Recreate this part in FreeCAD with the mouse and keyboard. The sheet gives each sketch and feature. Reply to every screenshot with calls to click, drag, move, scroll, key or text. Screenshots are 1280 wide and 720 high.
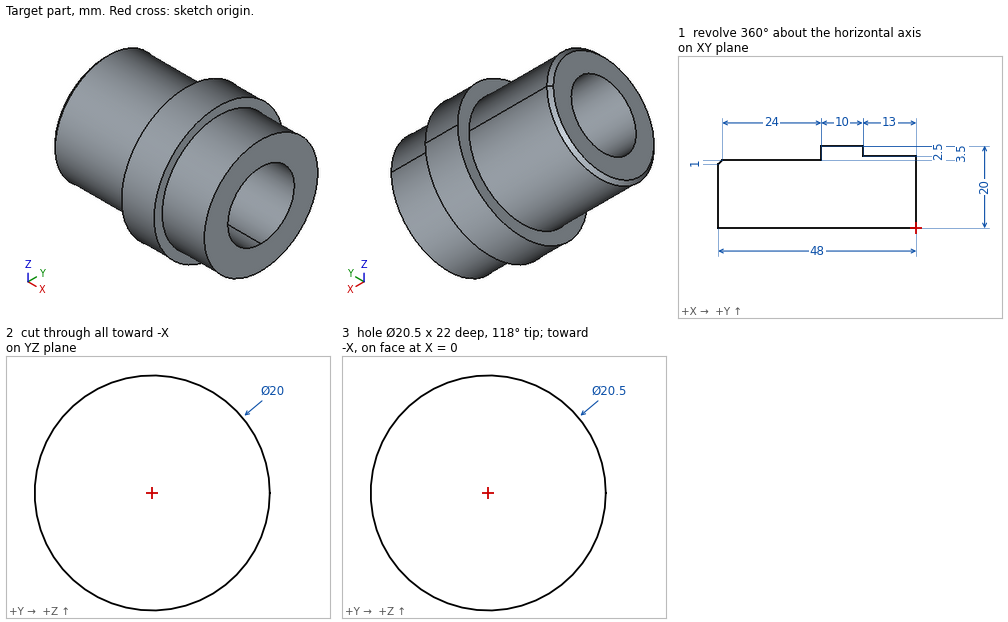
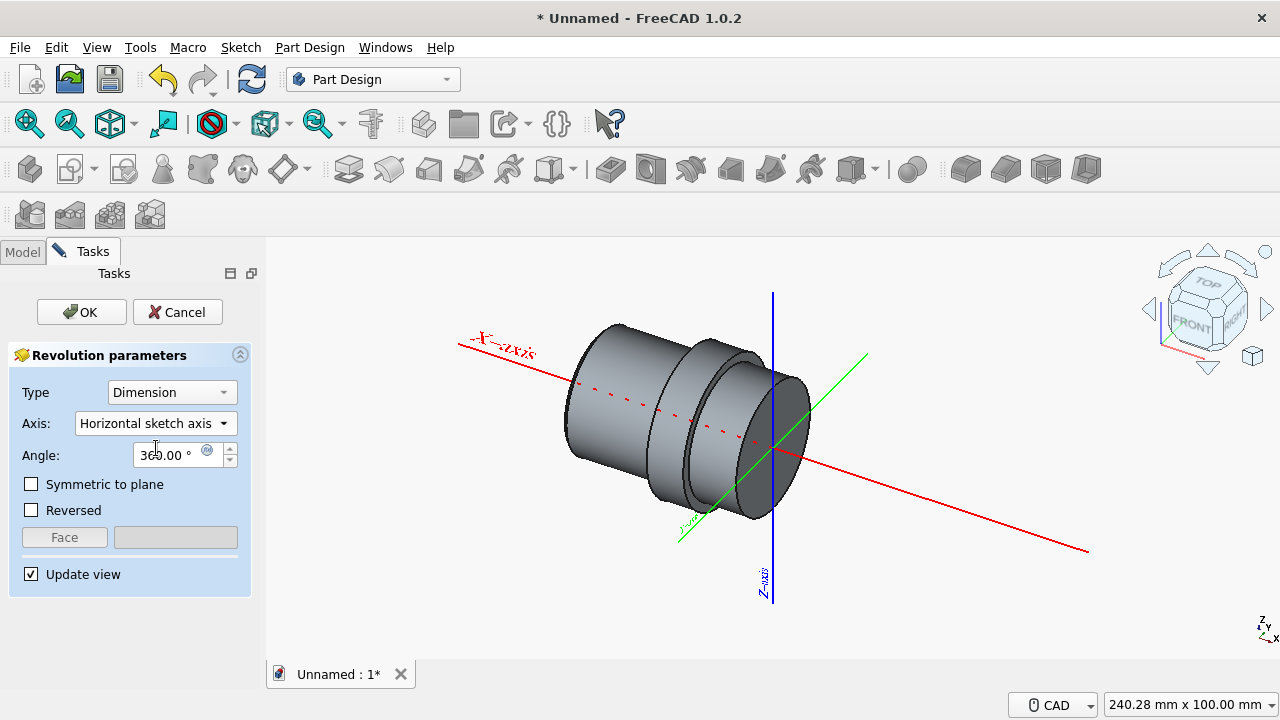
click(82, 312)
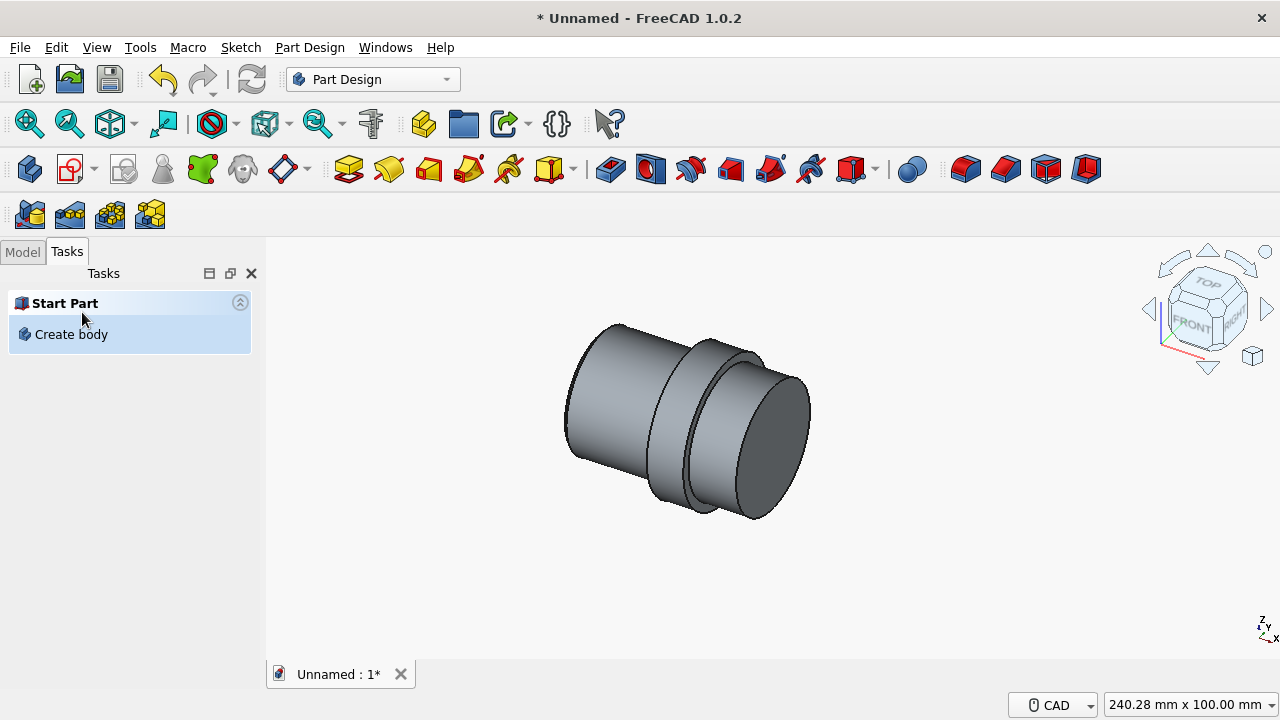
click(70, 170)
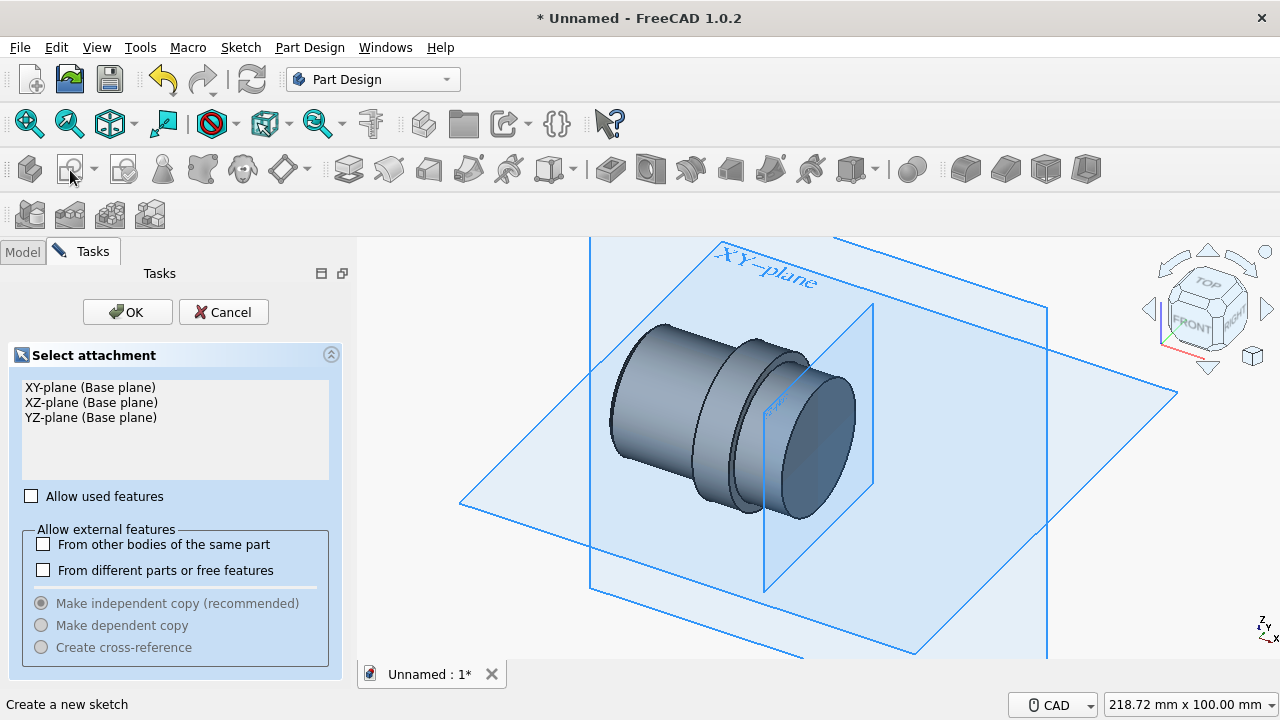
click(82, 418)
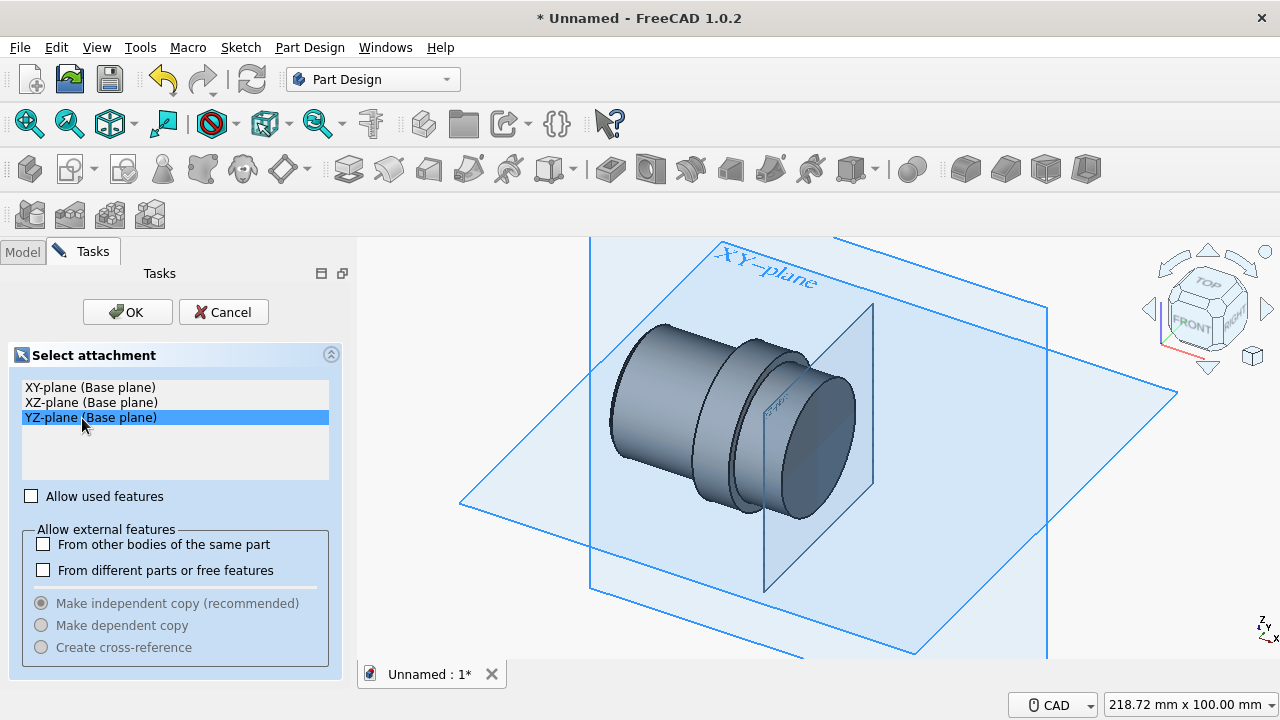
click(128, 312)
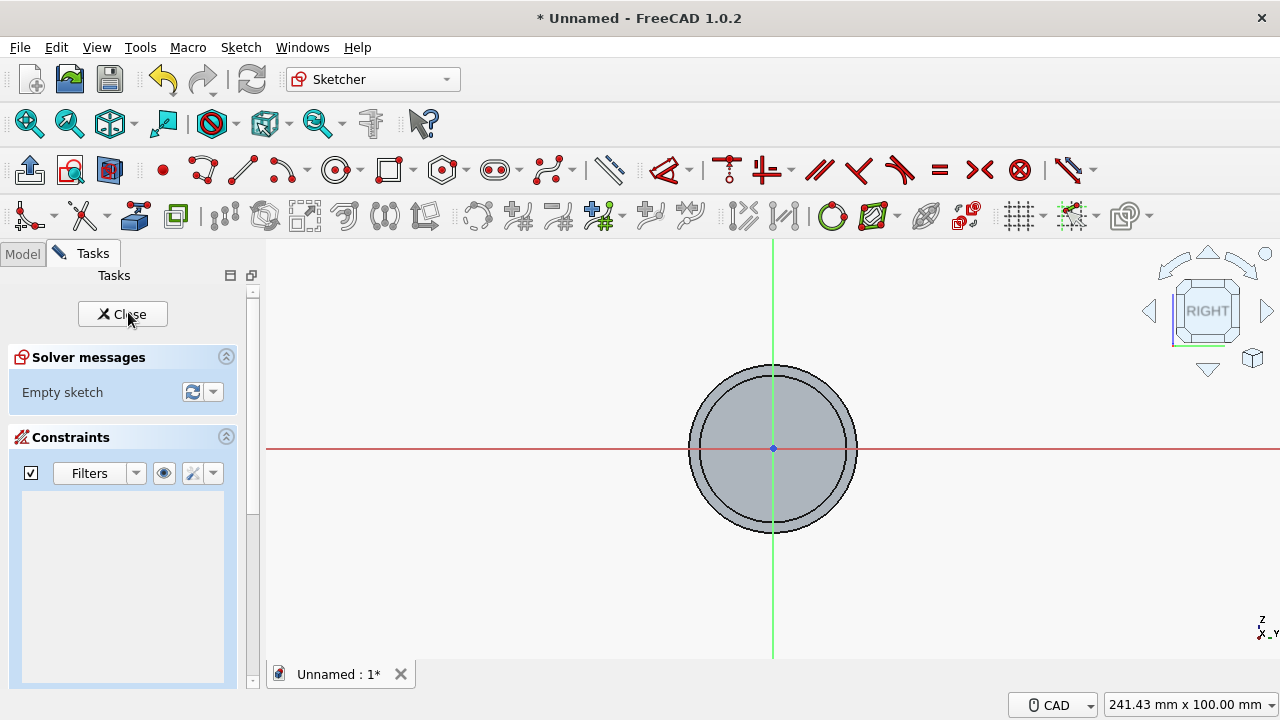
scroll(803, 449, up, 6)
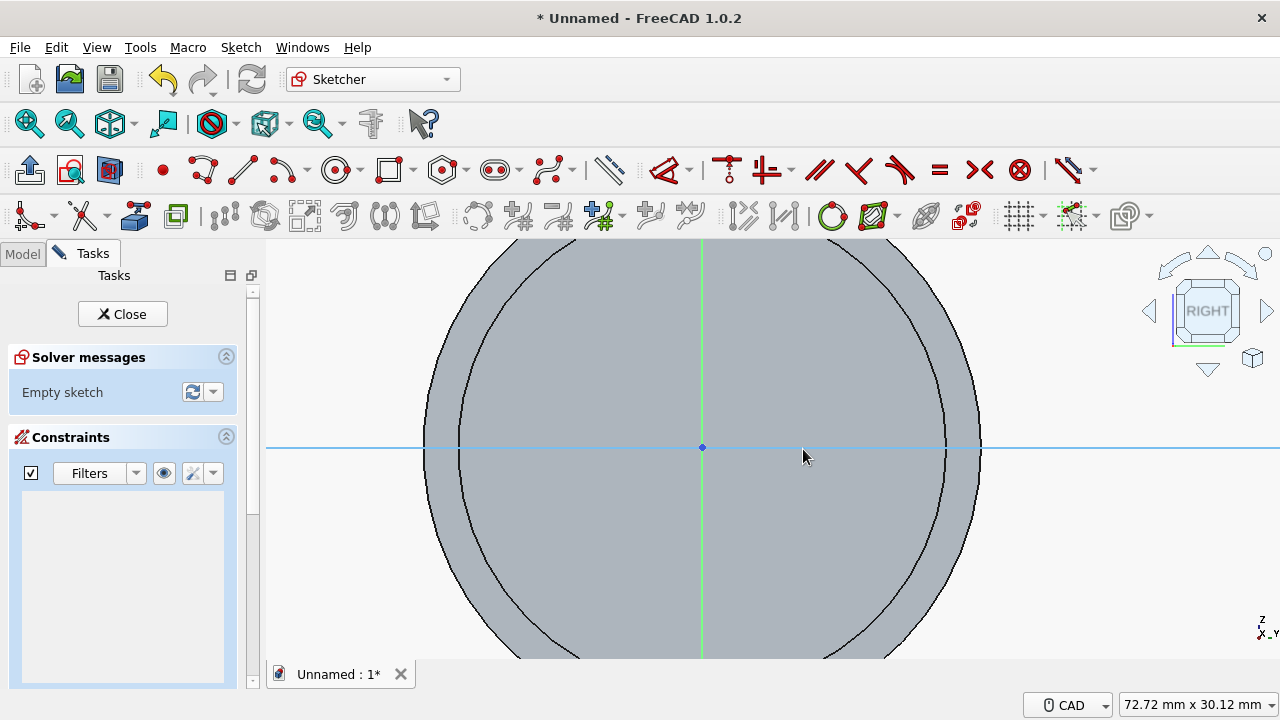
key(g)
key(c)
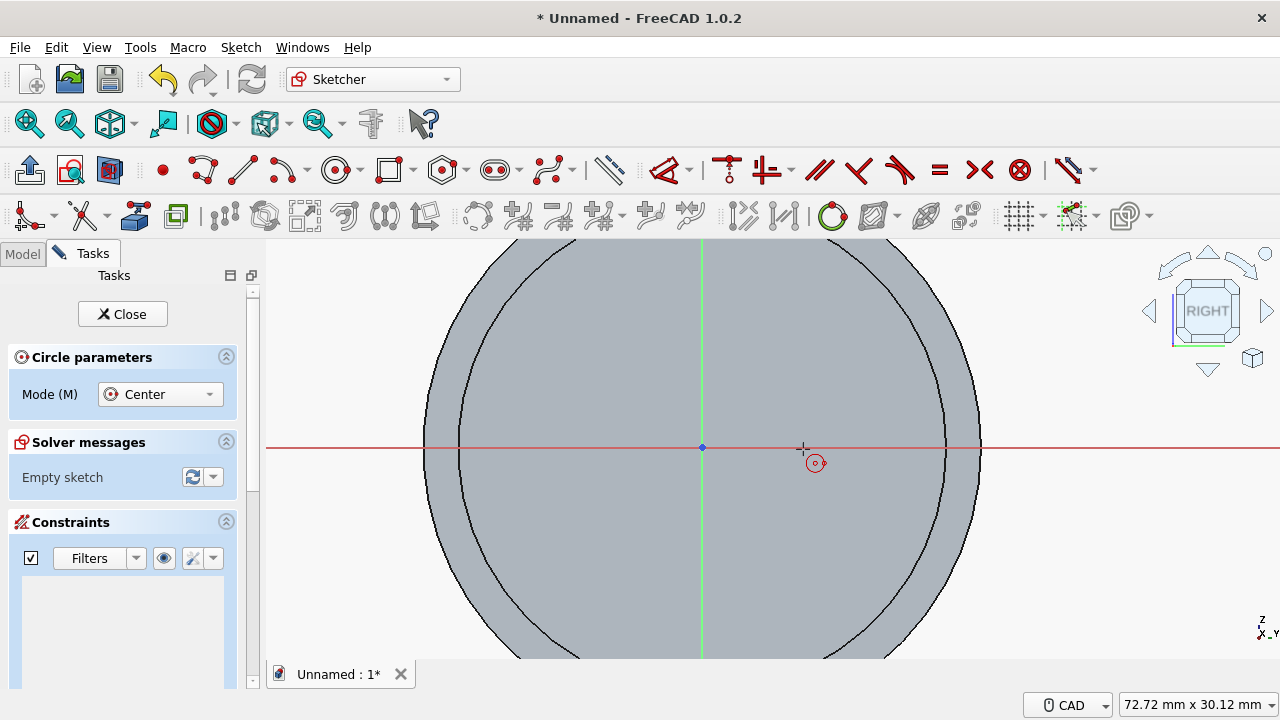
click(702, 448)
move(801, 349)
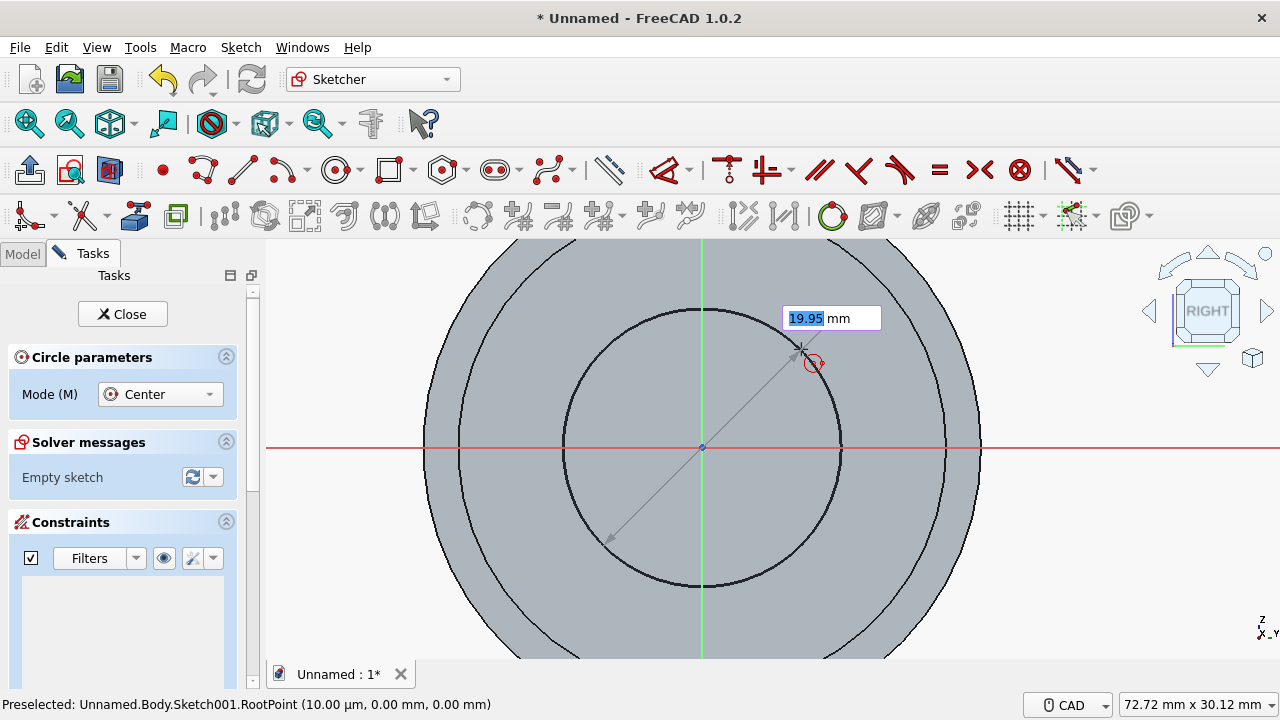
text(20)
key(Return)
key(Escape)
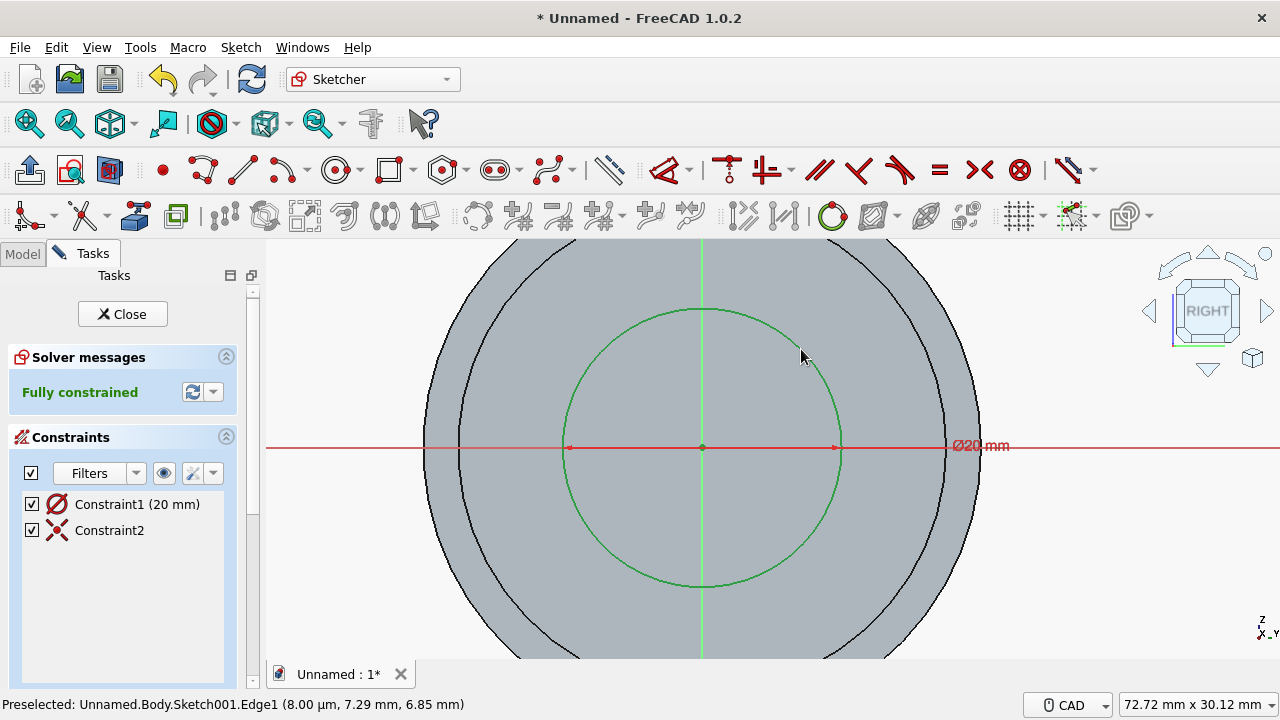
click(123, 314)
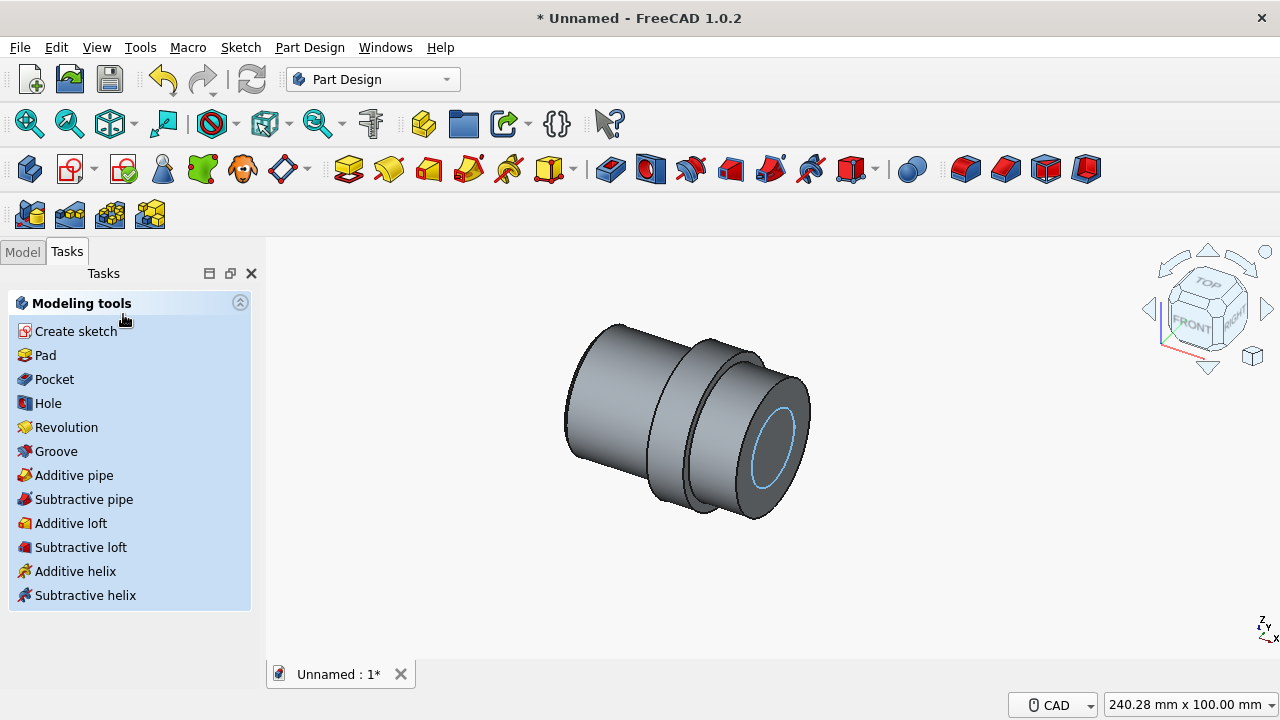
click(612, 170)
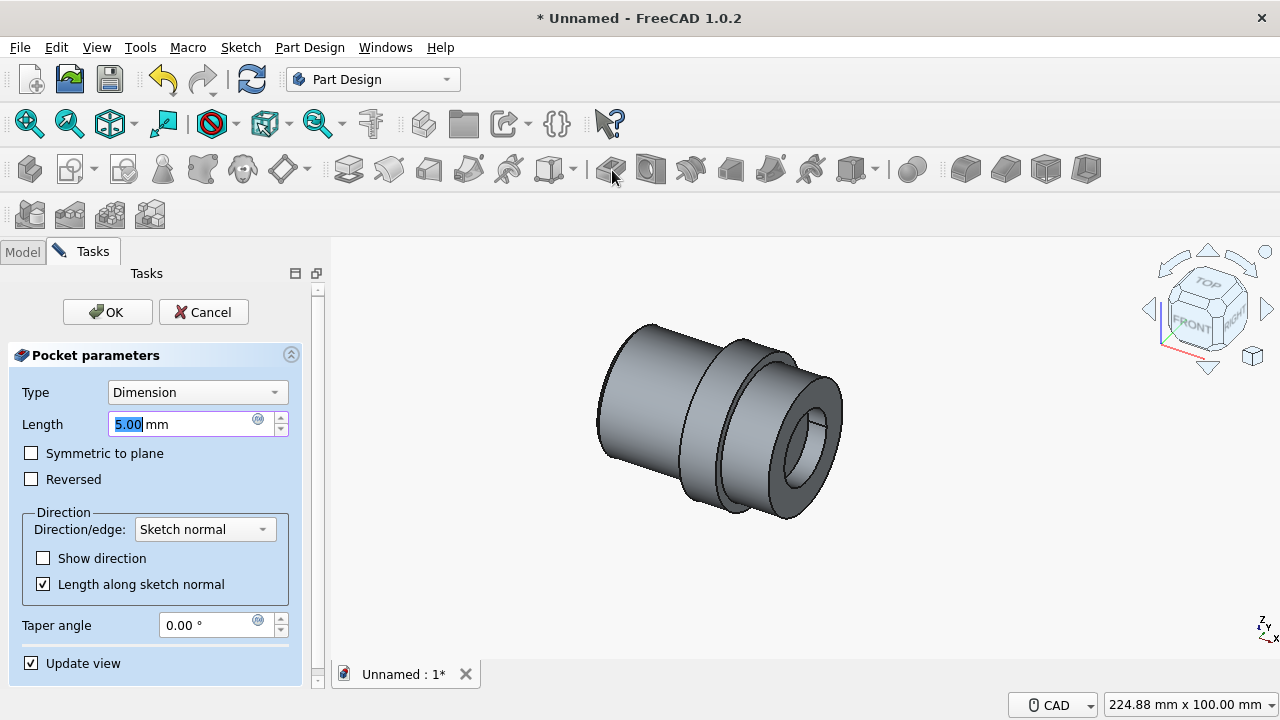
click(198, 392)